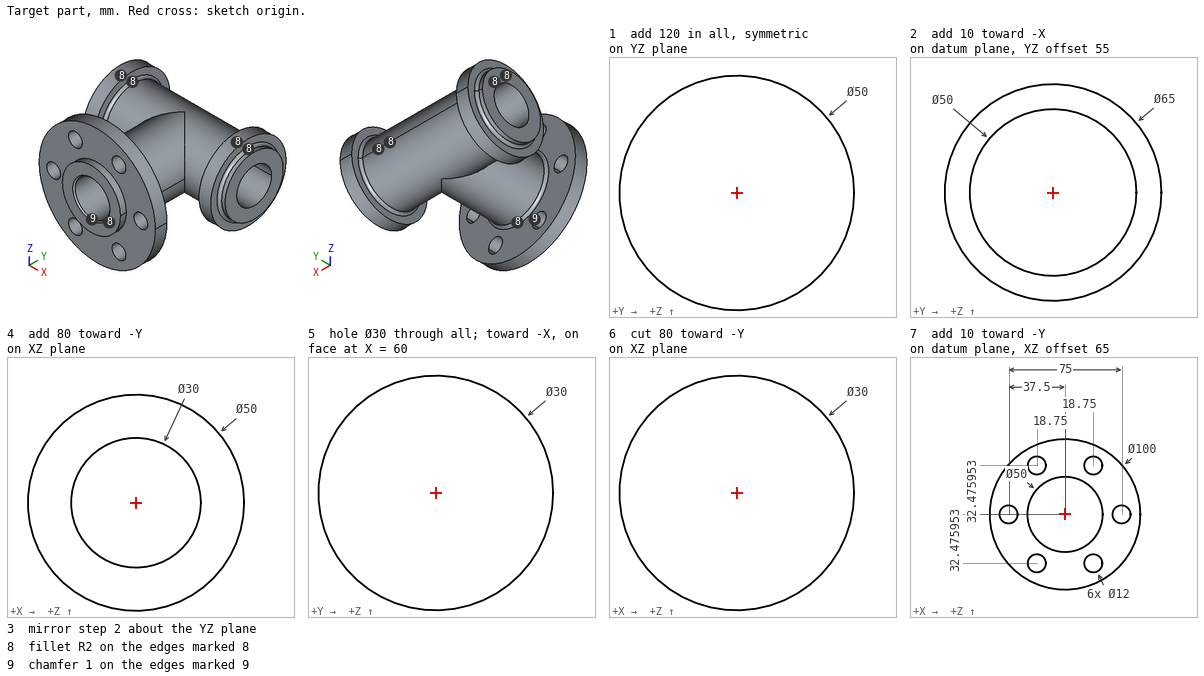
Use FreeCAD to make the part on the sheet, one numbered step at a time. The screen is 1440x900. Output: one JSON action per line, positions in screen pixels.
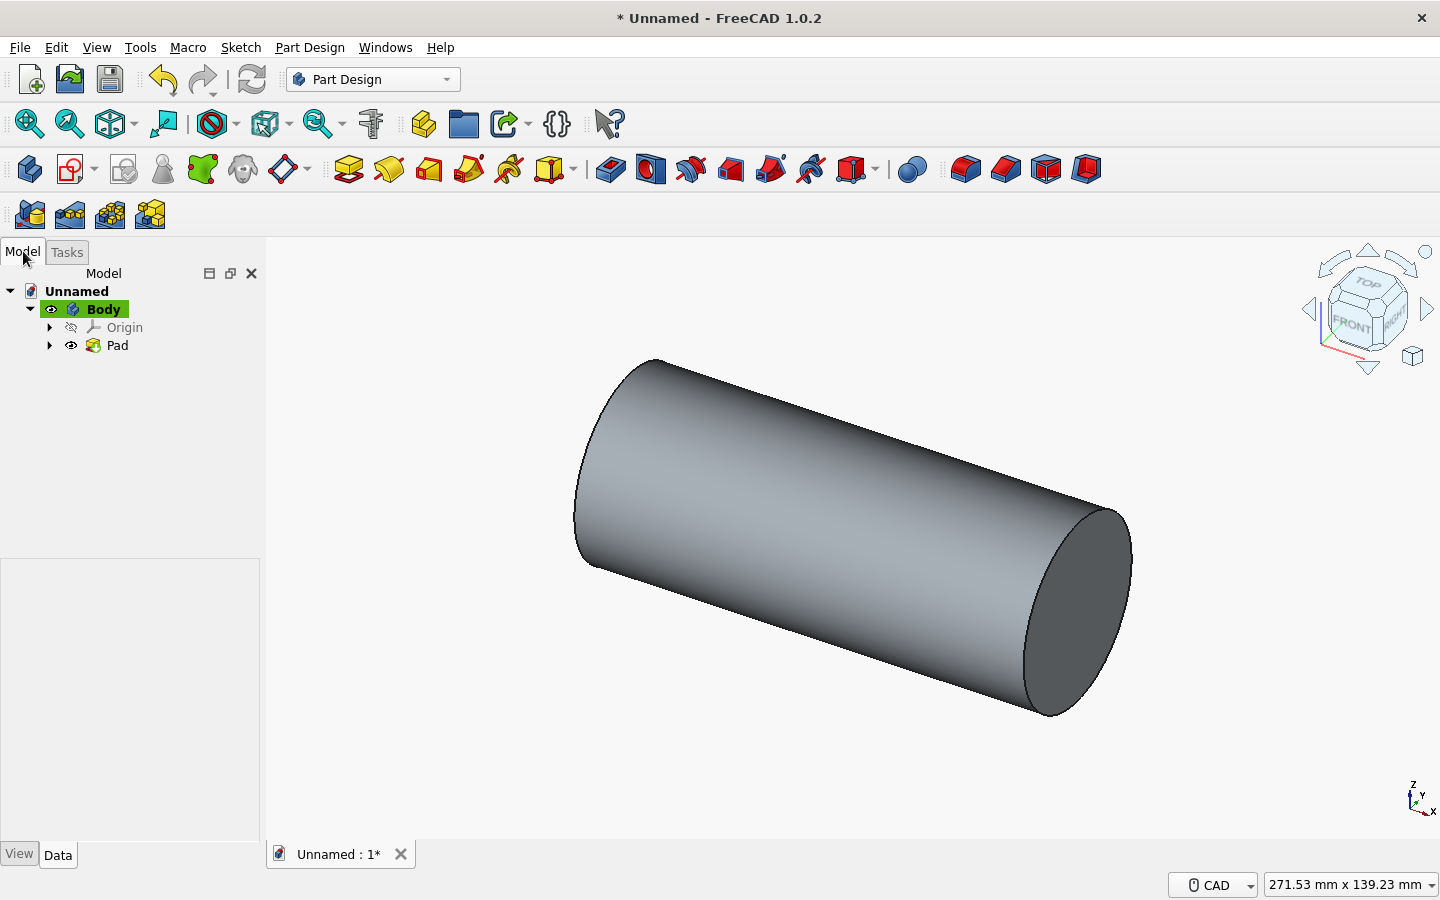
{"action": "left_click", "coordinate": [50, 327]}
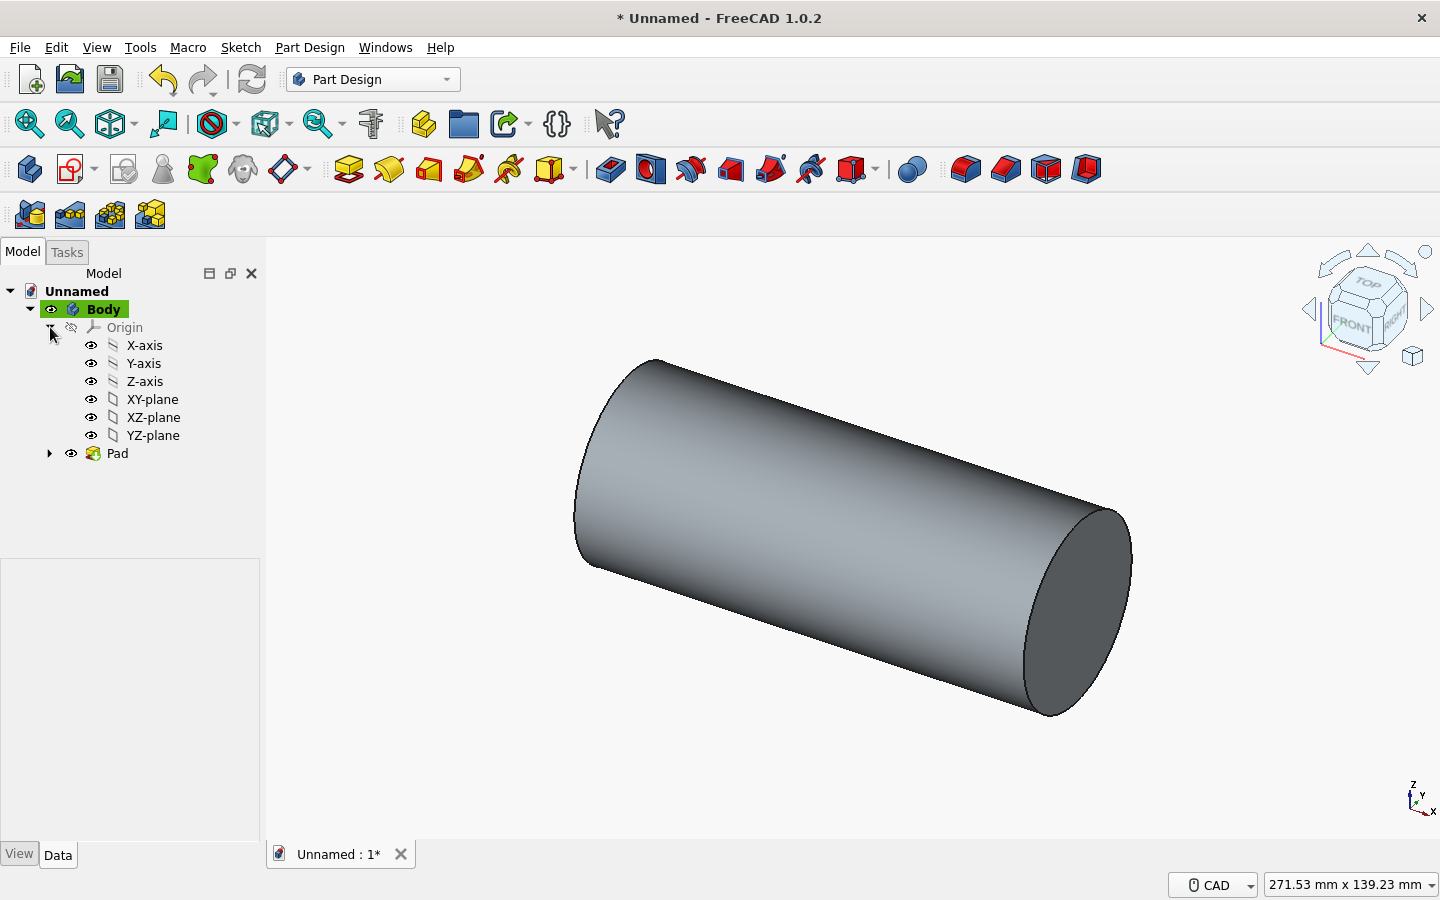
{"action": "left_click", "coordinate": [136, 435]}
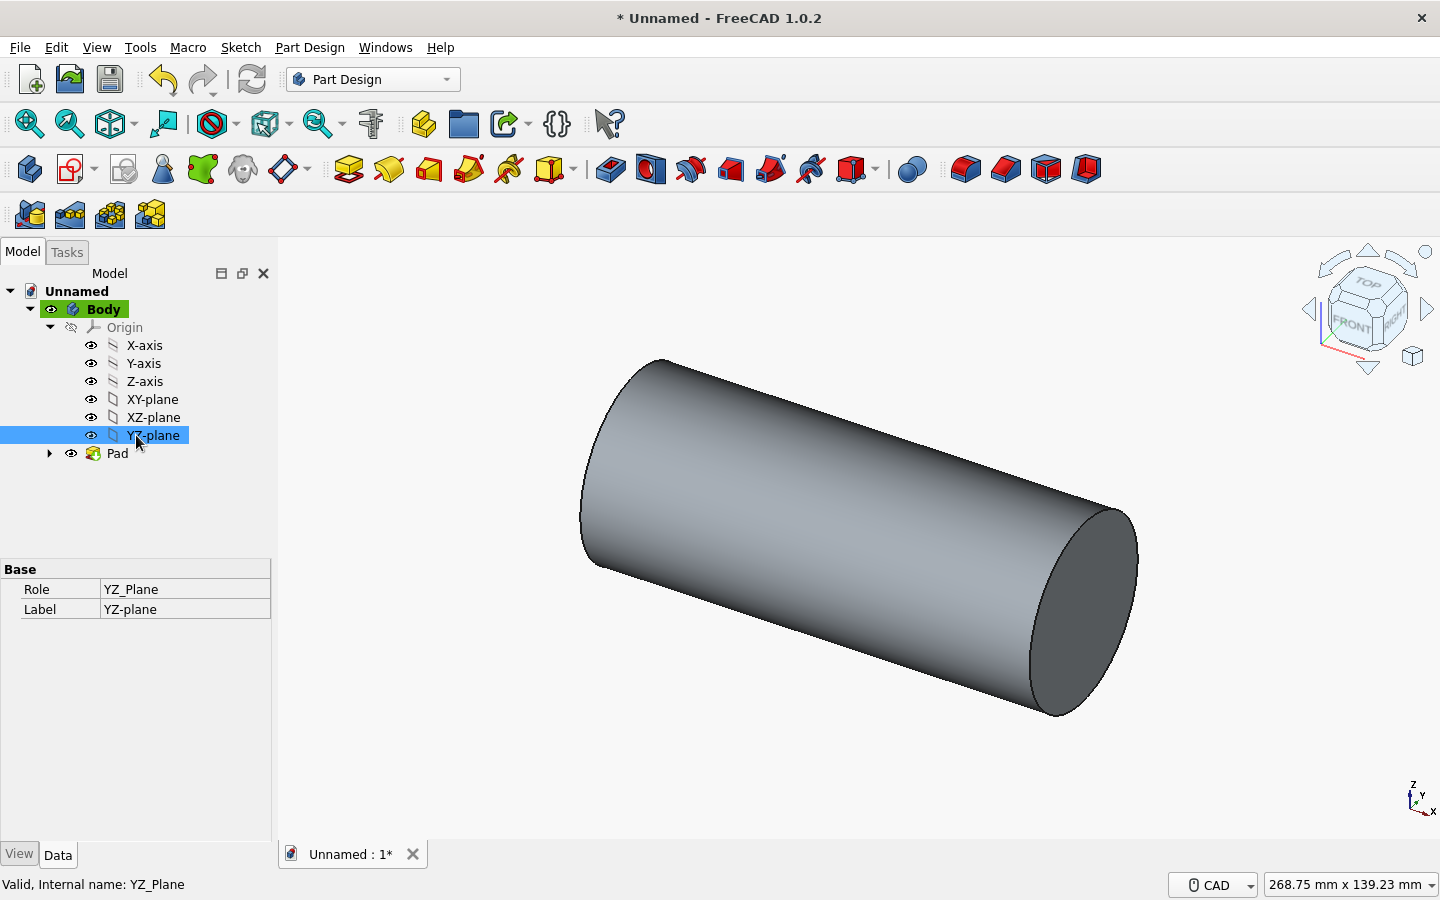
{"action": "left_click", "coordinate": [284, 170]}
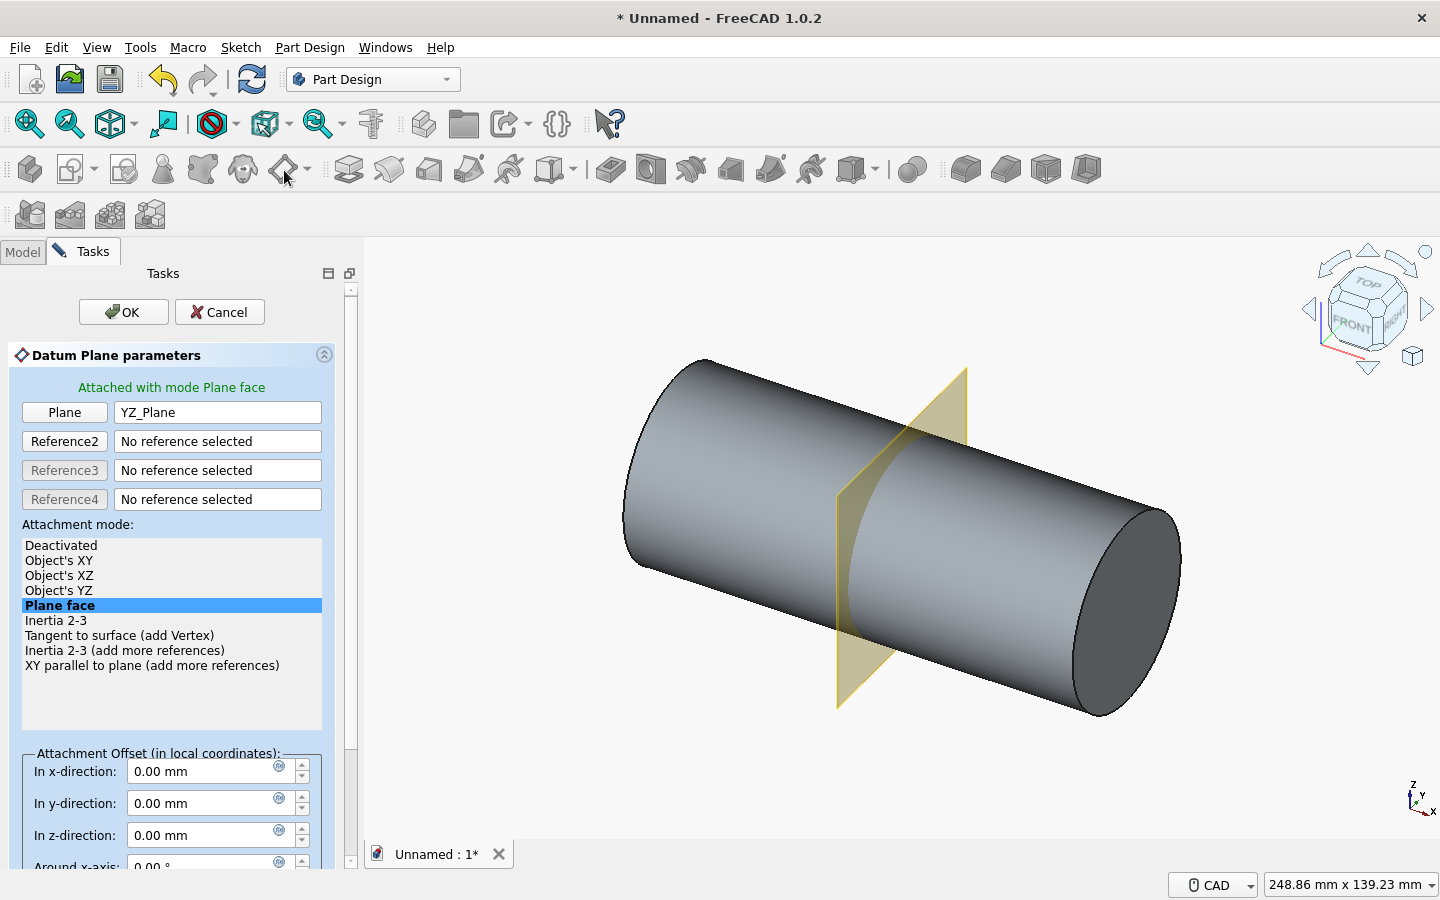
{"action": "triple_click", "coordinate": [210, 835]}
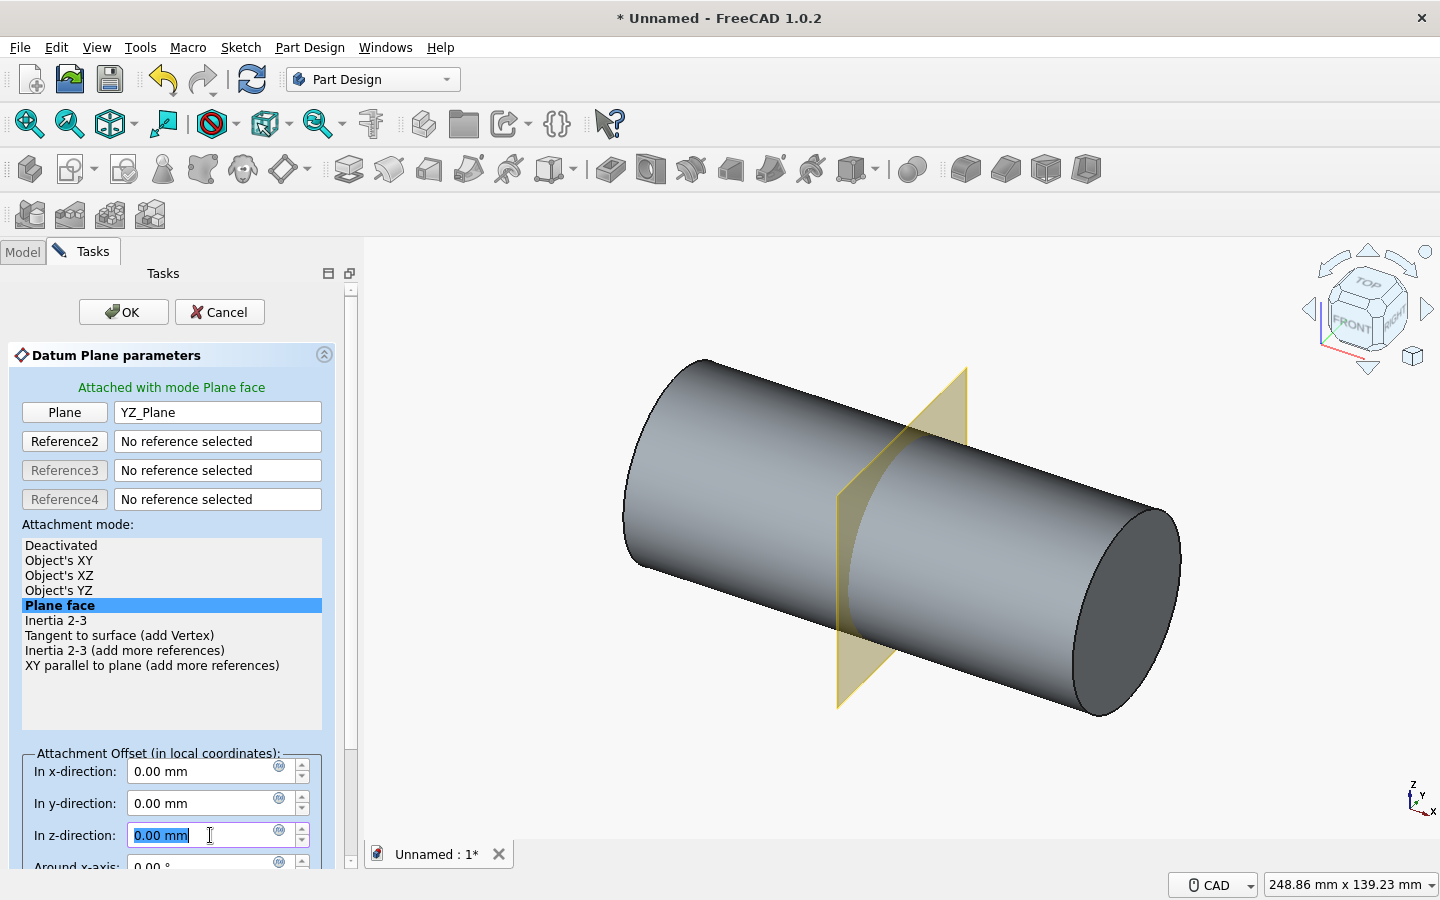
{"action": "type", "text": "55"}
{"action": "key", "text": "Tab"}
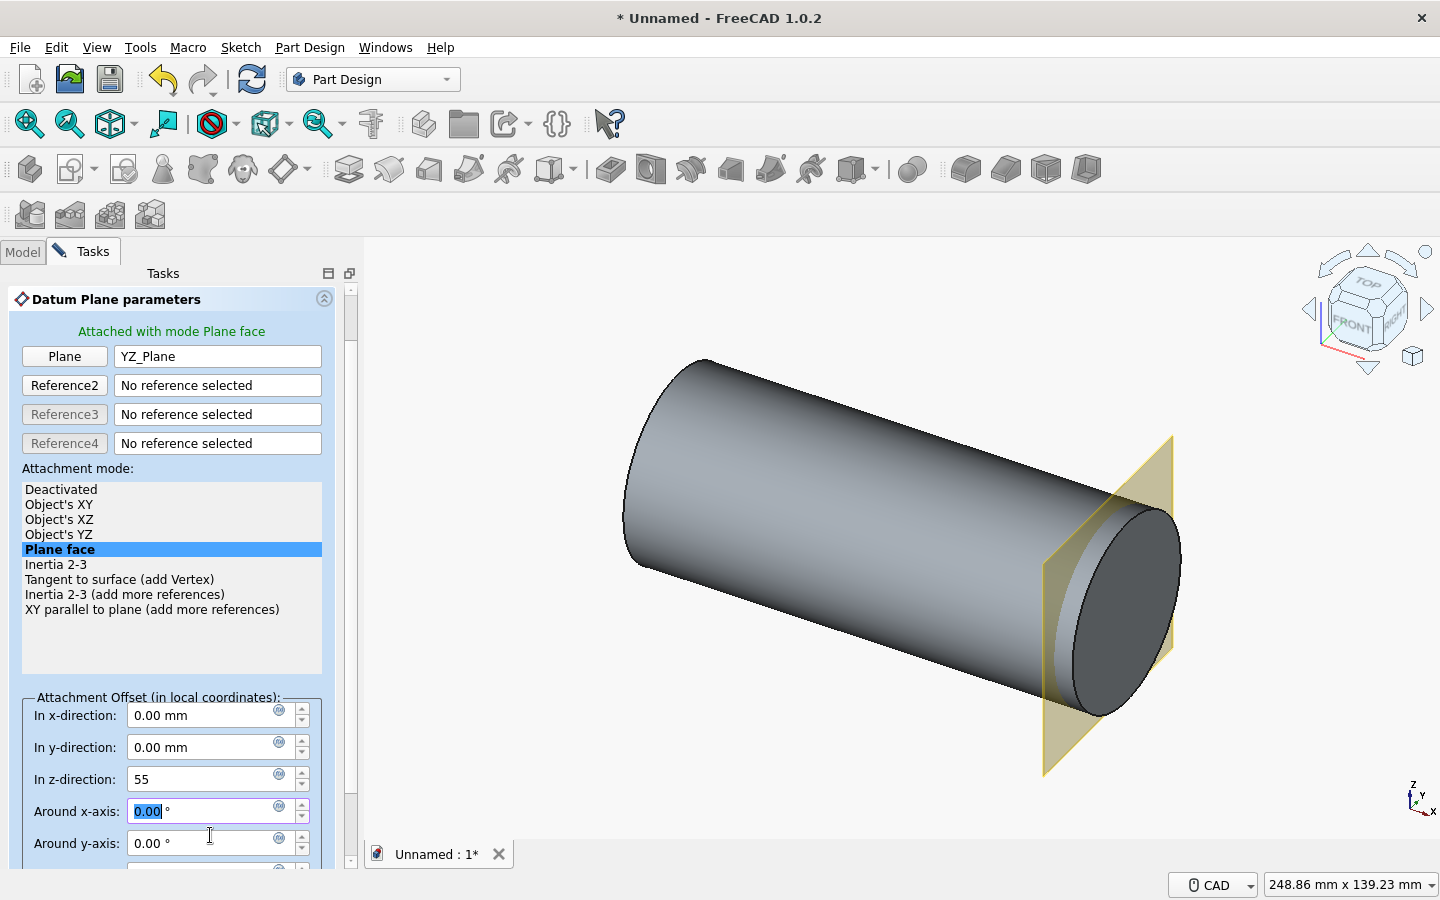
{"action": "scroll", "coordinate": [351, 576], "scroll_direction": "up", "scroll_amount": 2}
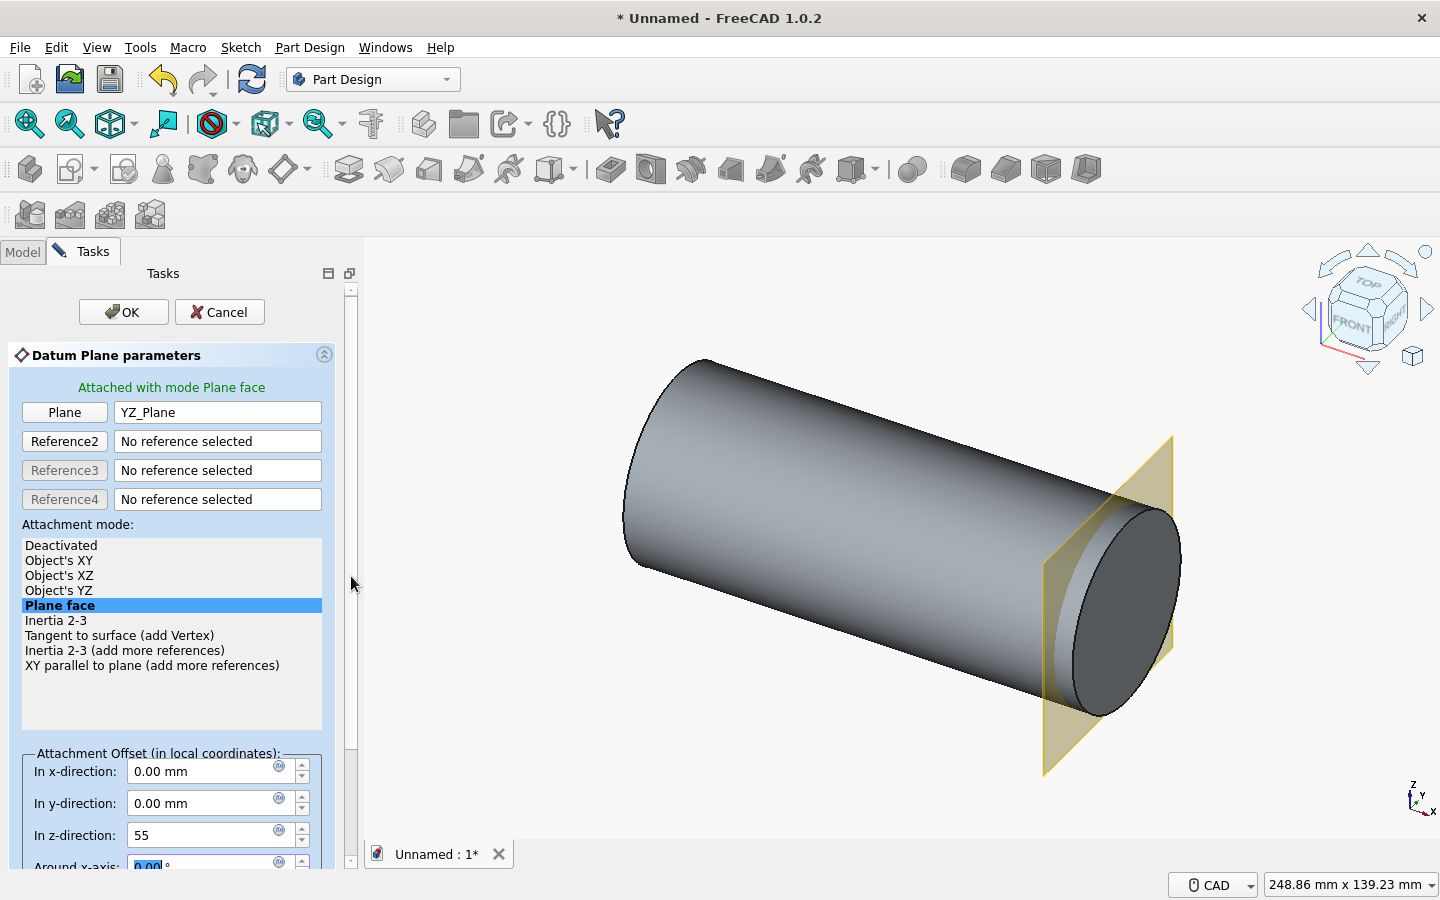
{"action": "left_click", "coordinate": [124, 312]}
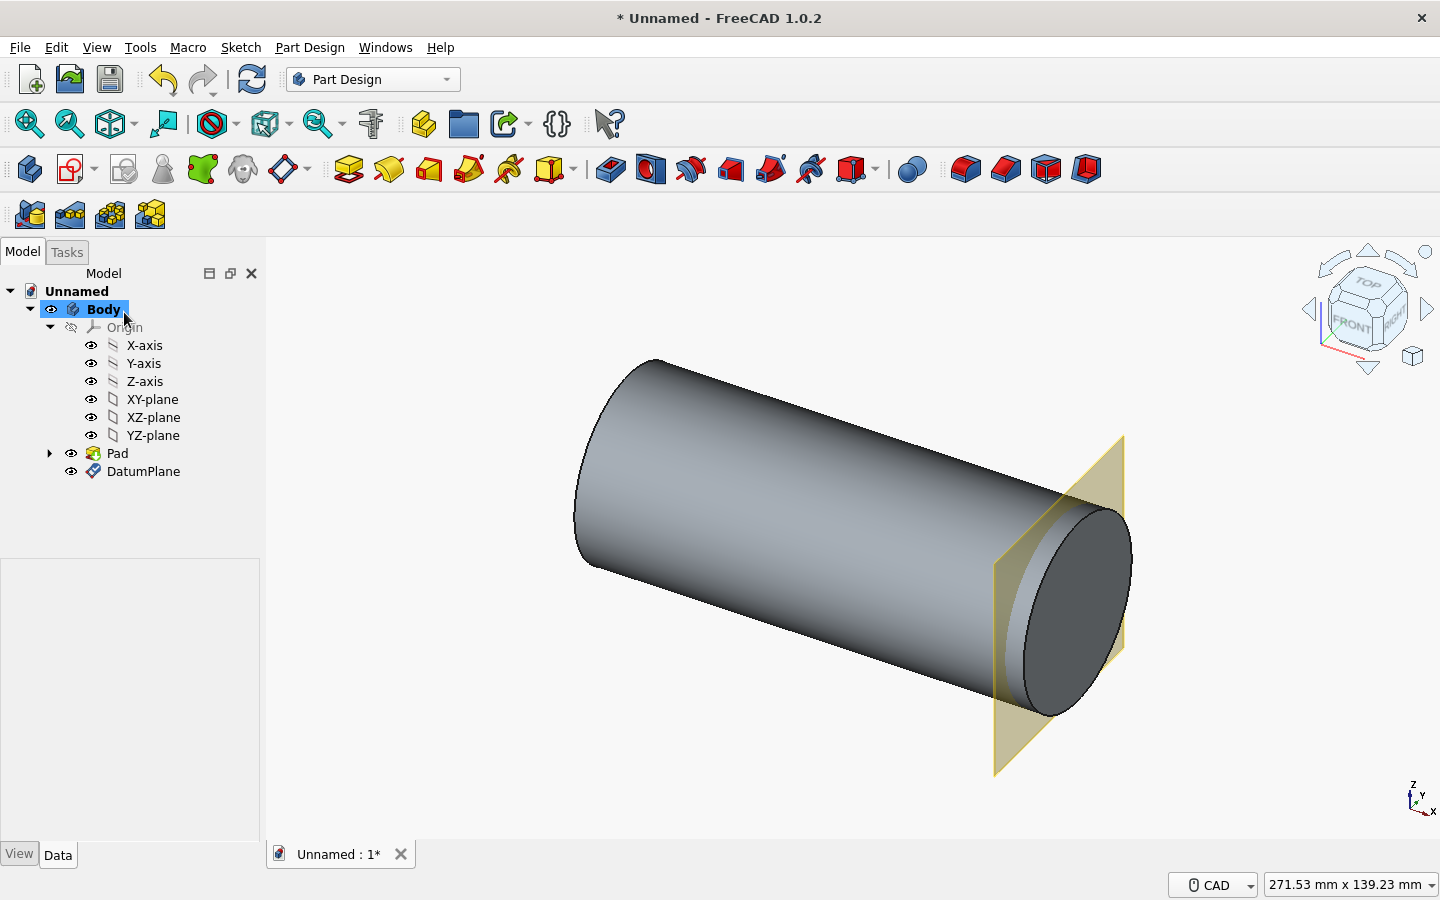
{"action": "left_click", "coordinate": [116, 471]}